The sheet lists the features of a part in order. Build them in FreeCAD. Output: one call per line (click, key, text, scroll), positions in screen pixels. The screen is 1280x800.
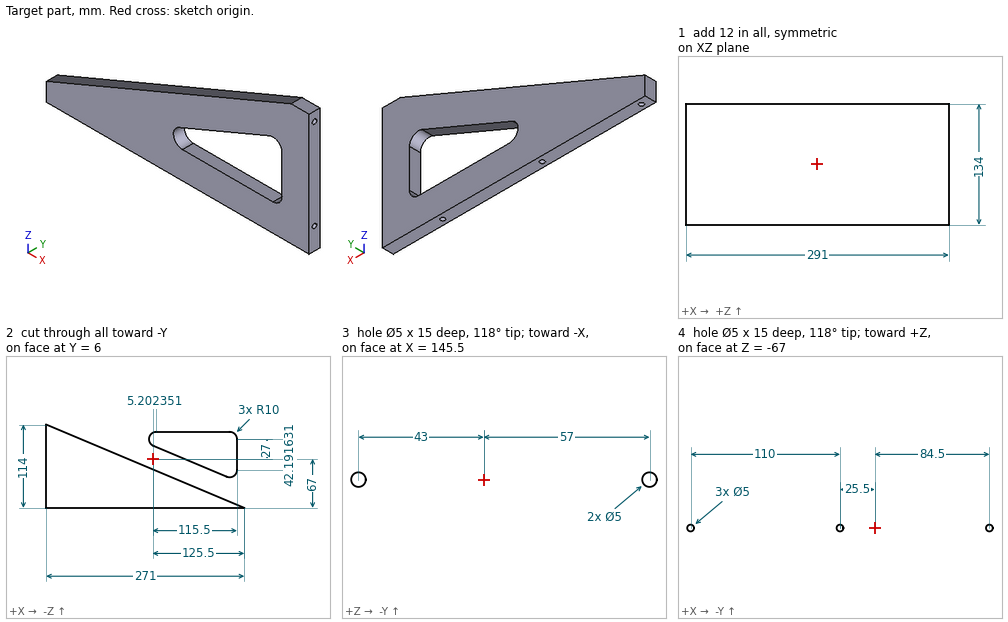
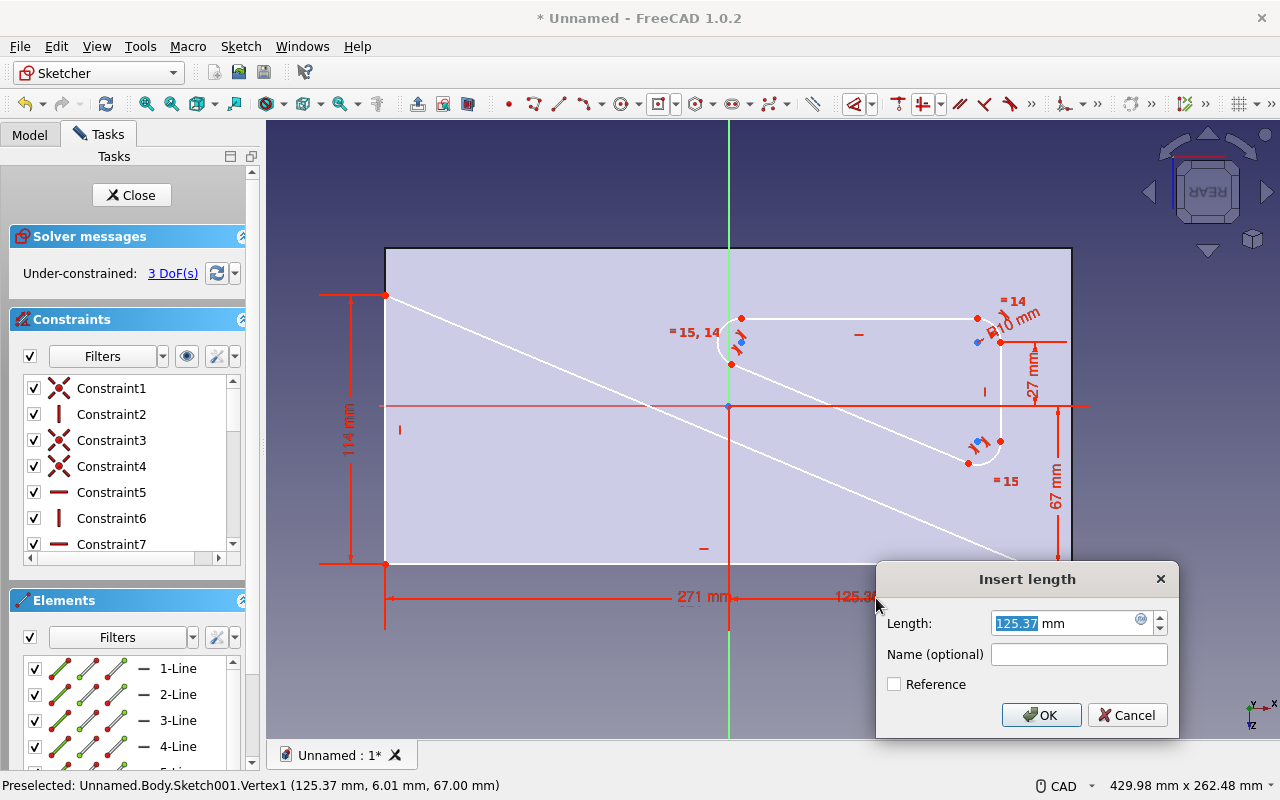
text(125.5)
key(Return)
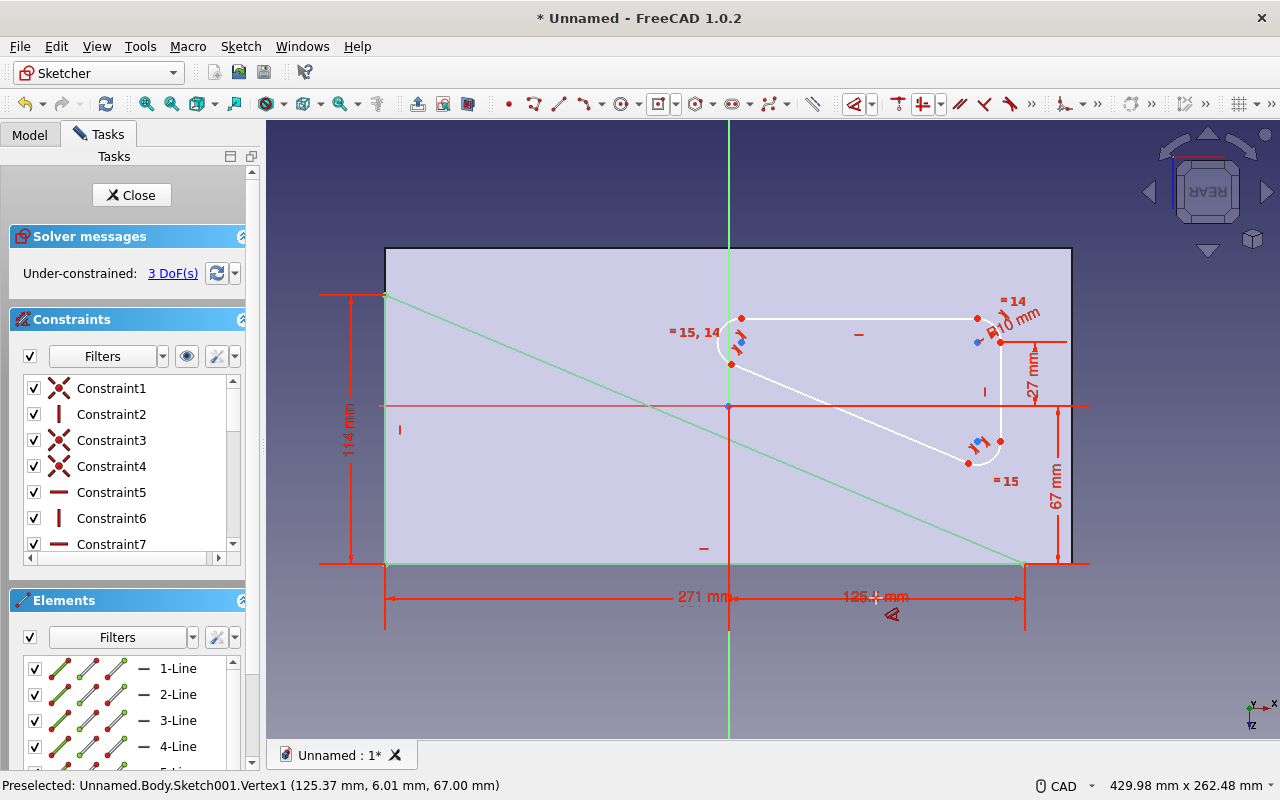
click(1001, 441)
click(865, 372)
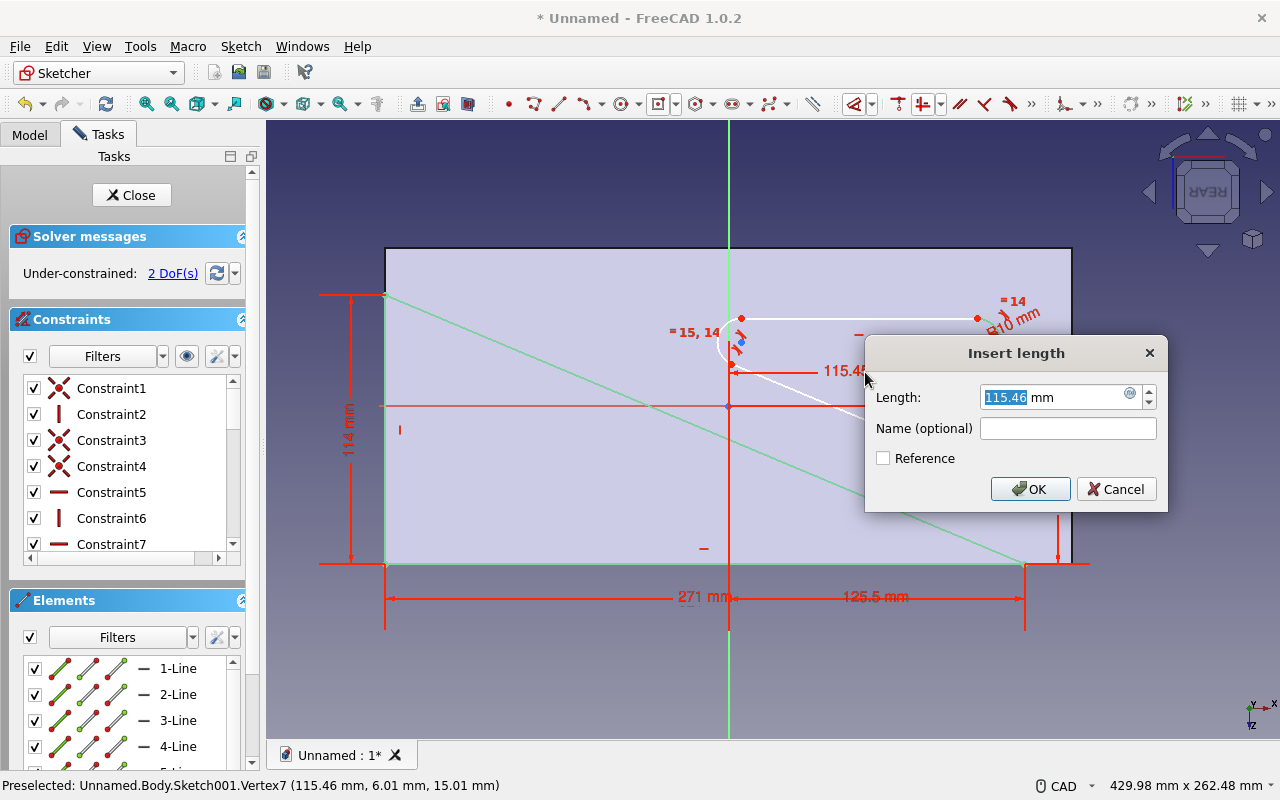
text(115.5)
key(Return)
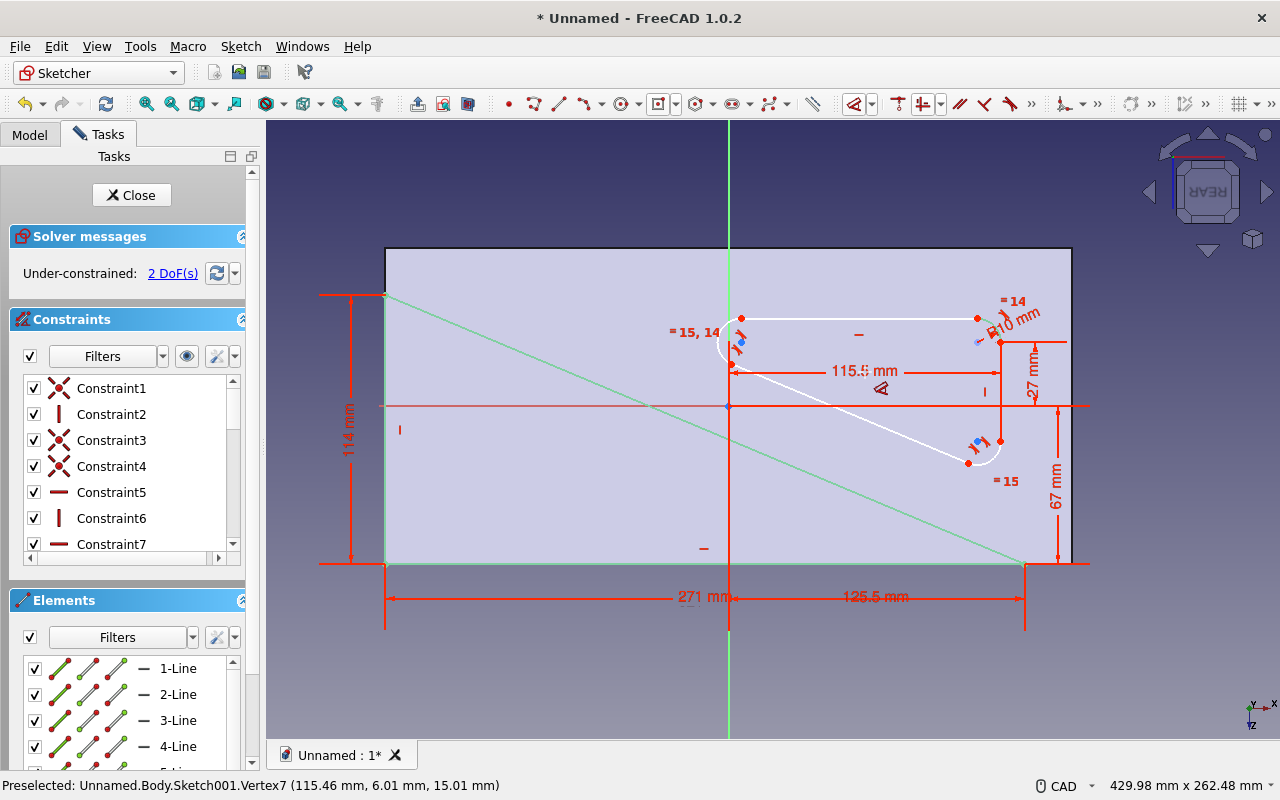
click(1001, 372)
click(1035, 427)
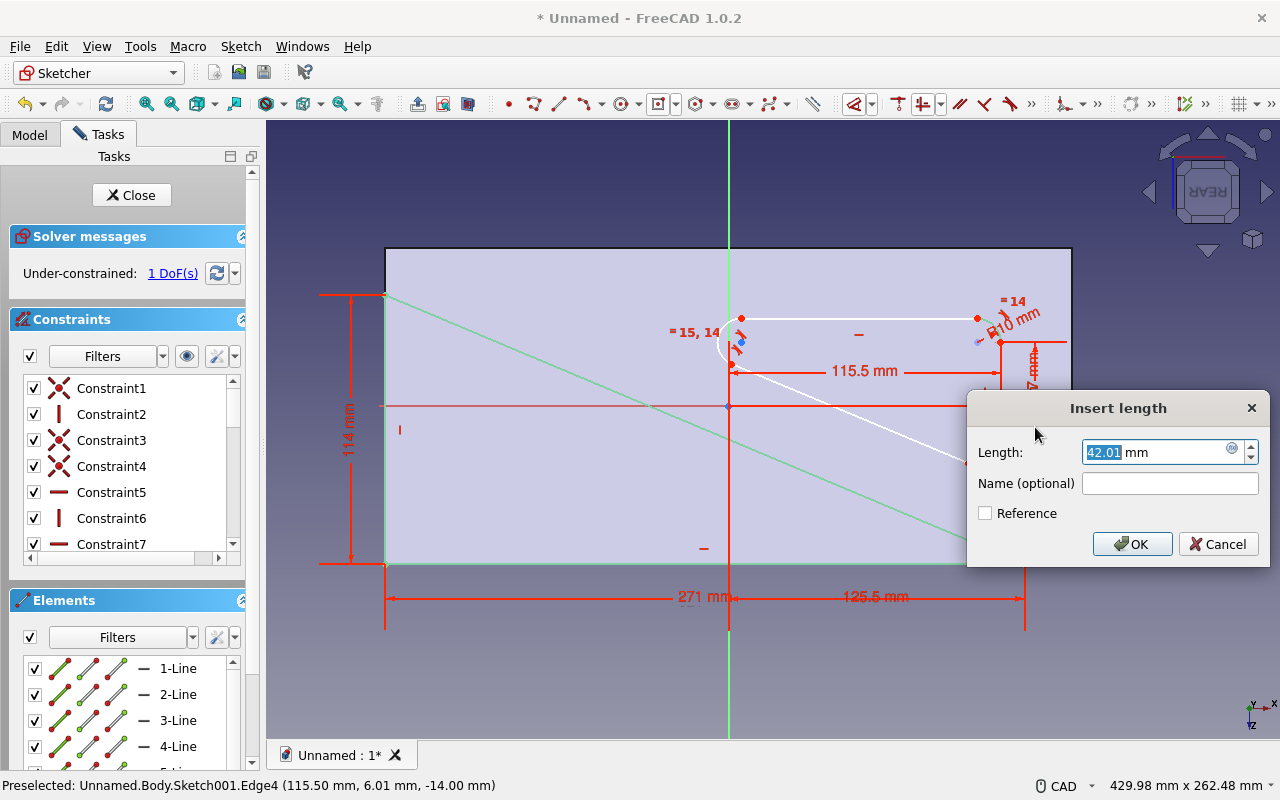
text(42.191631)
key(Return)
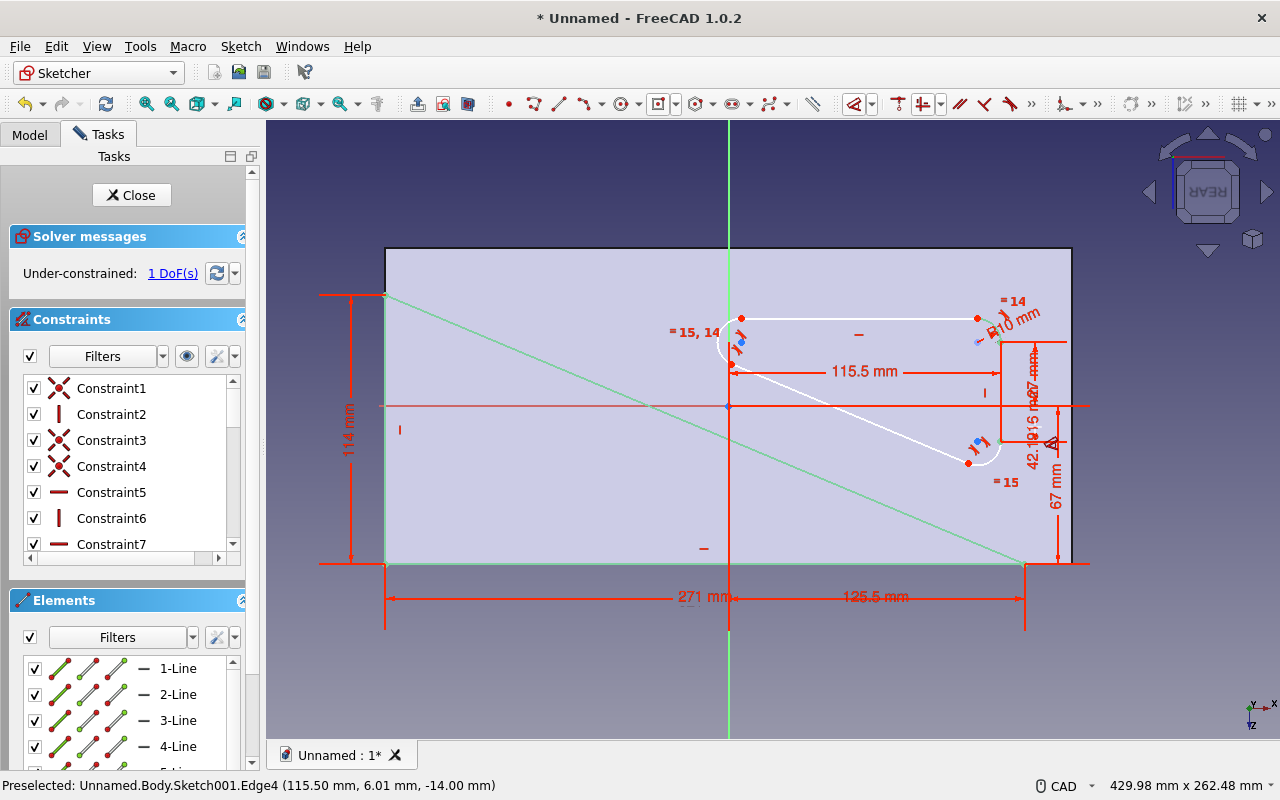
scroll(741, 319, up, 6)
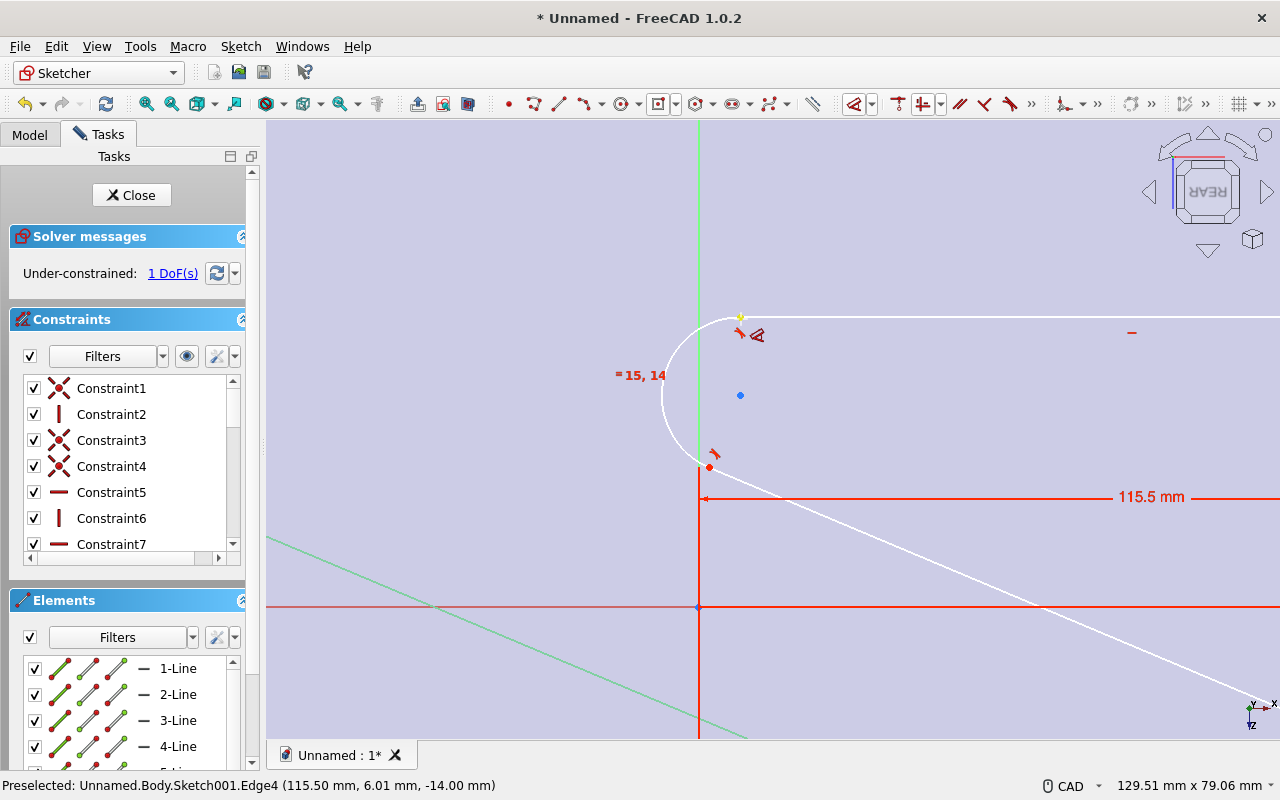
click(740, 317)
click(719, 283)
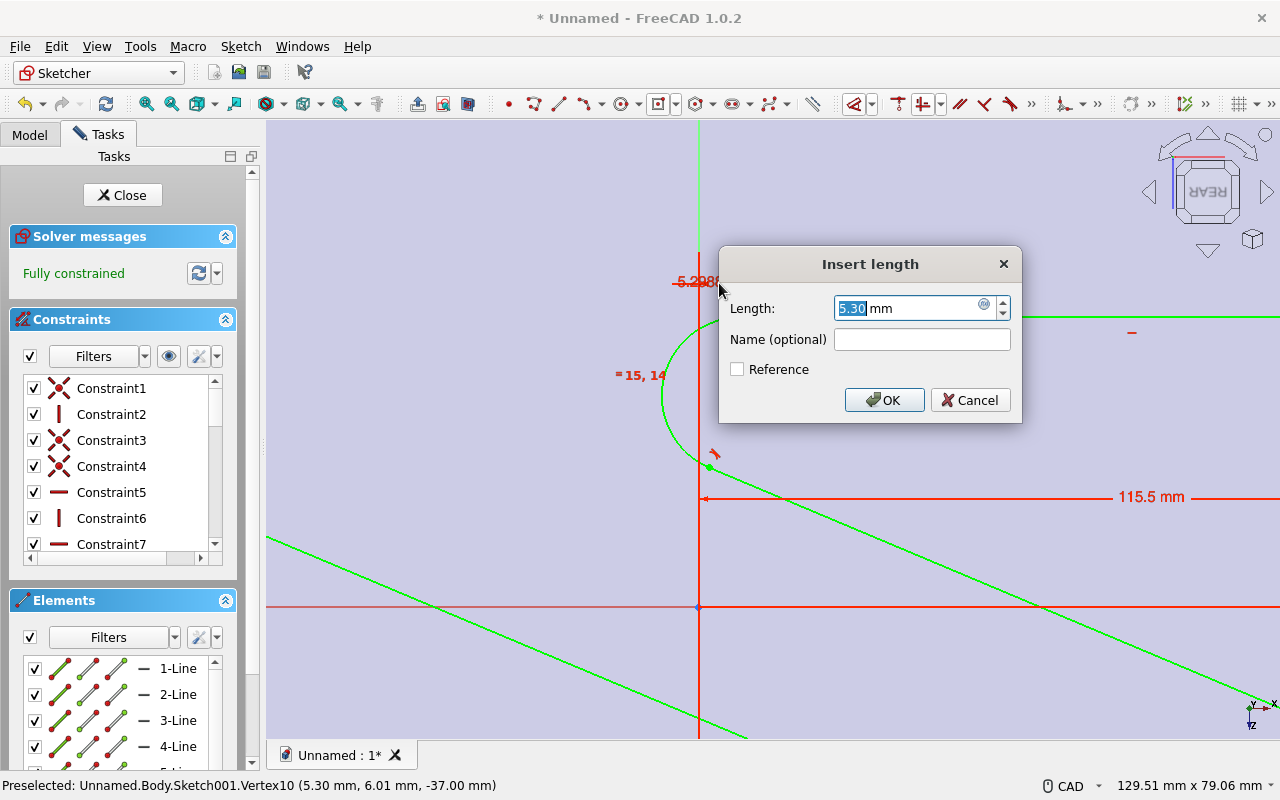
text(5.202351)
key(Return)
key(Escape)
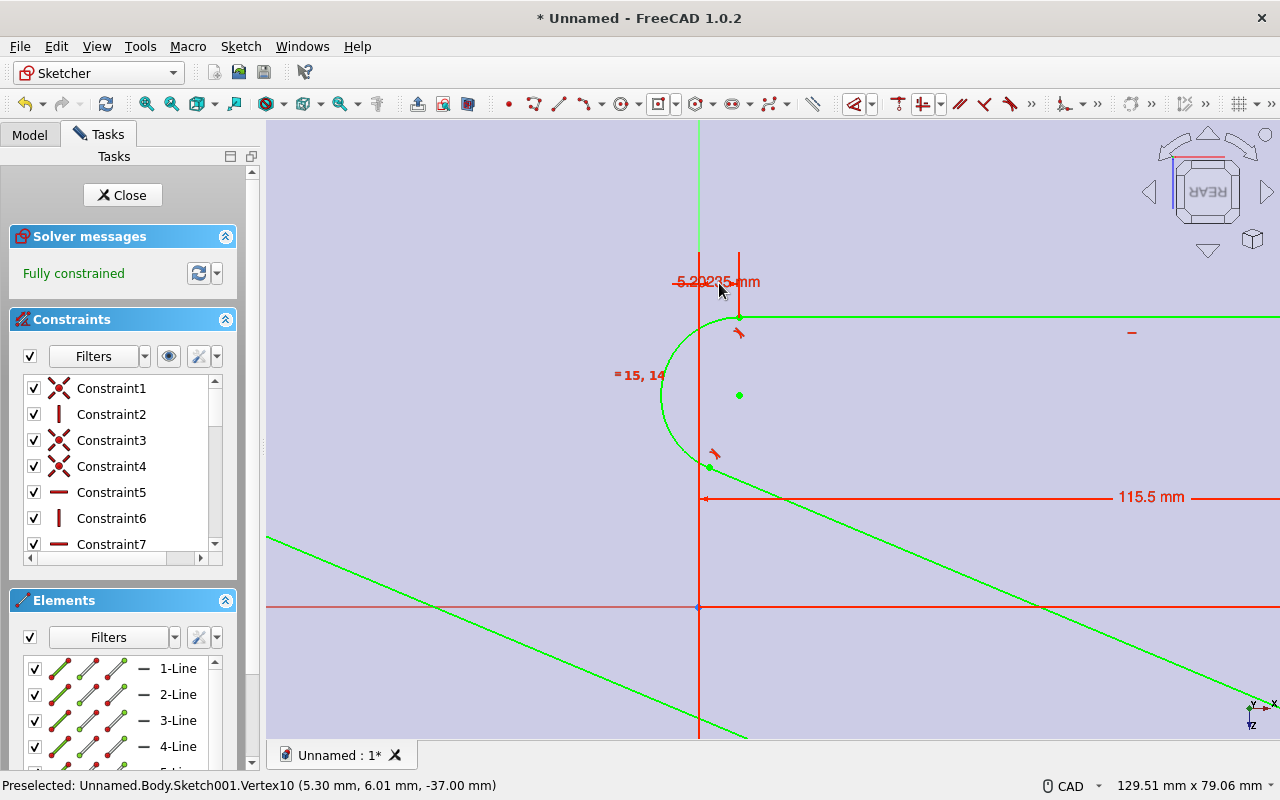
click(123, 195)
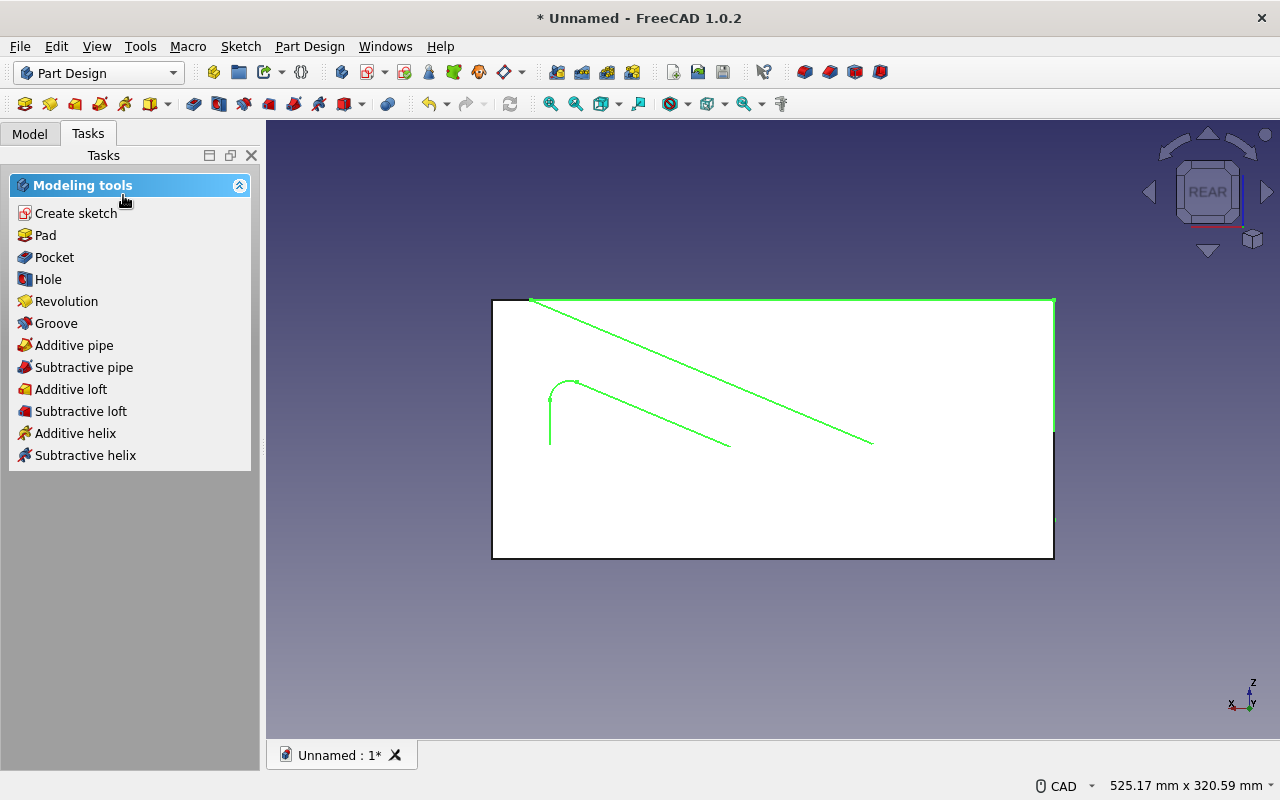
click(194, 104)